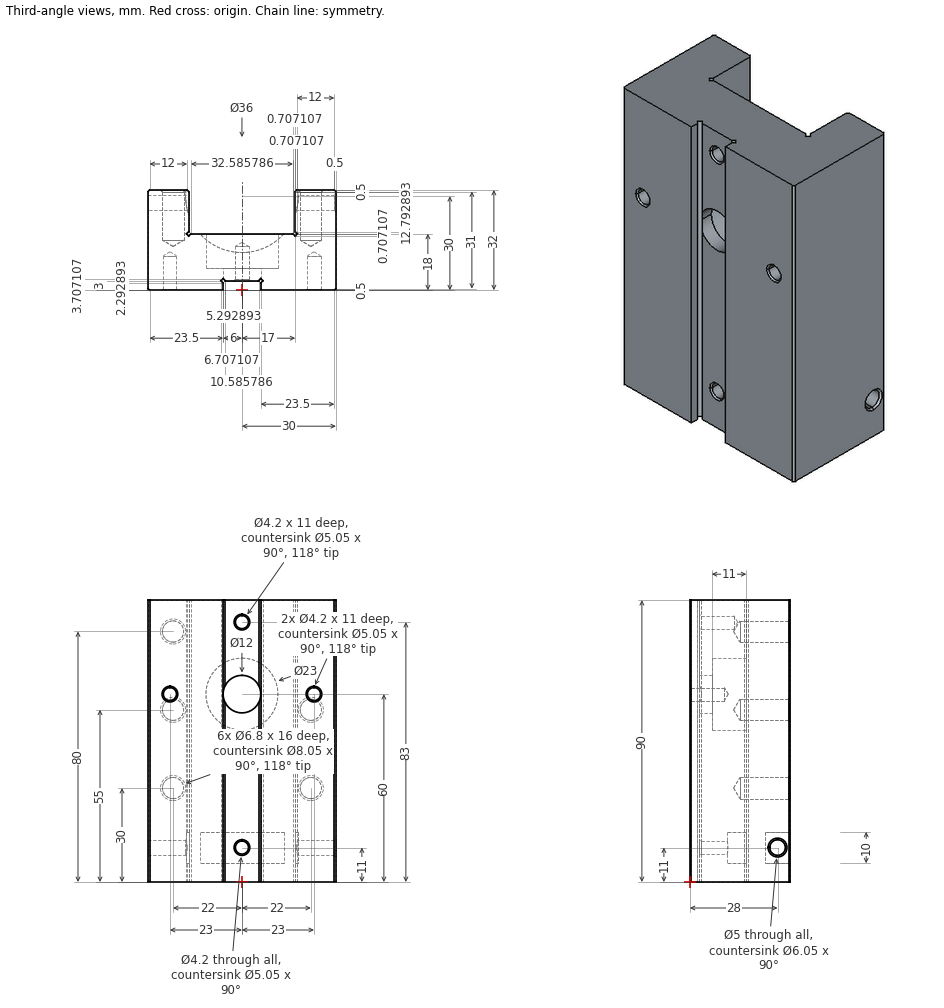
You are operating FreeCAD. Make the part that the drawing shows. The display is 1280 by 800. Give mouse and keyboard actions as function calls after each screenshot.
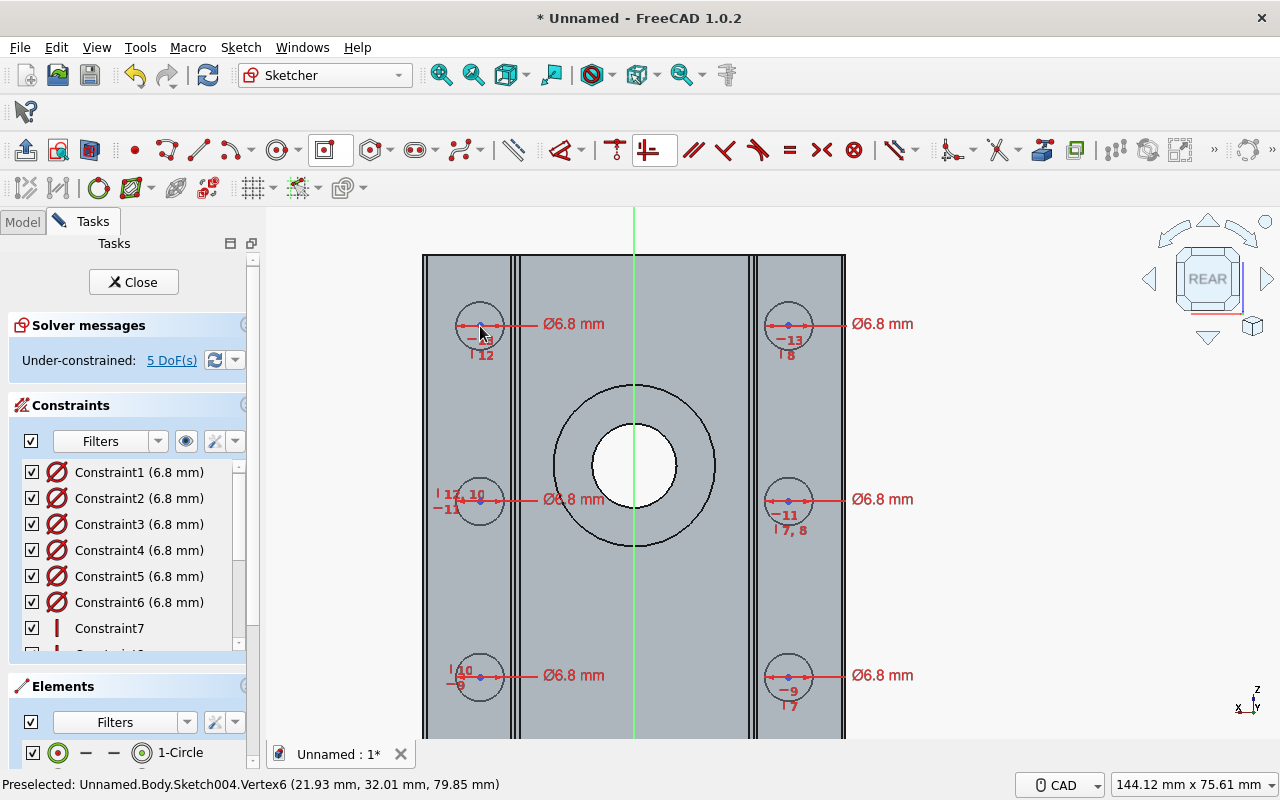
click(560, 150)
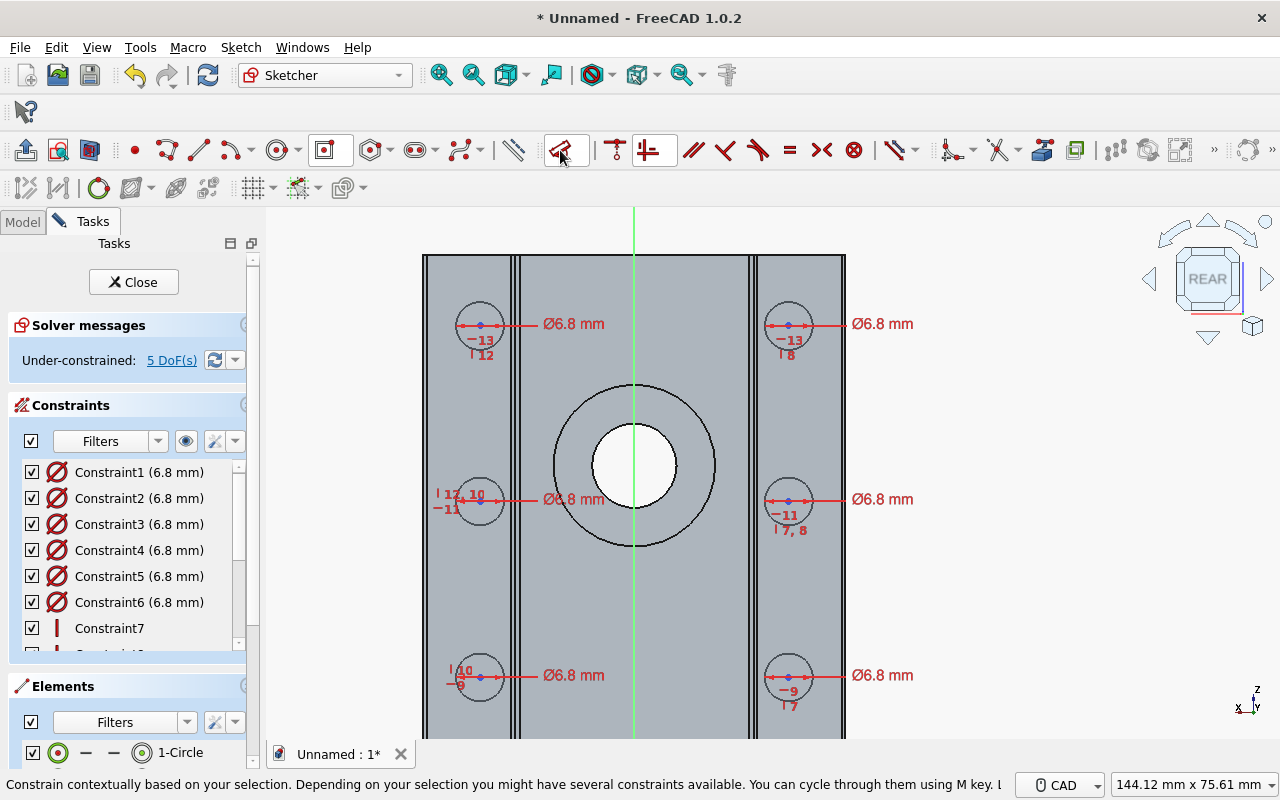
click(789, 677)
click(712, 643)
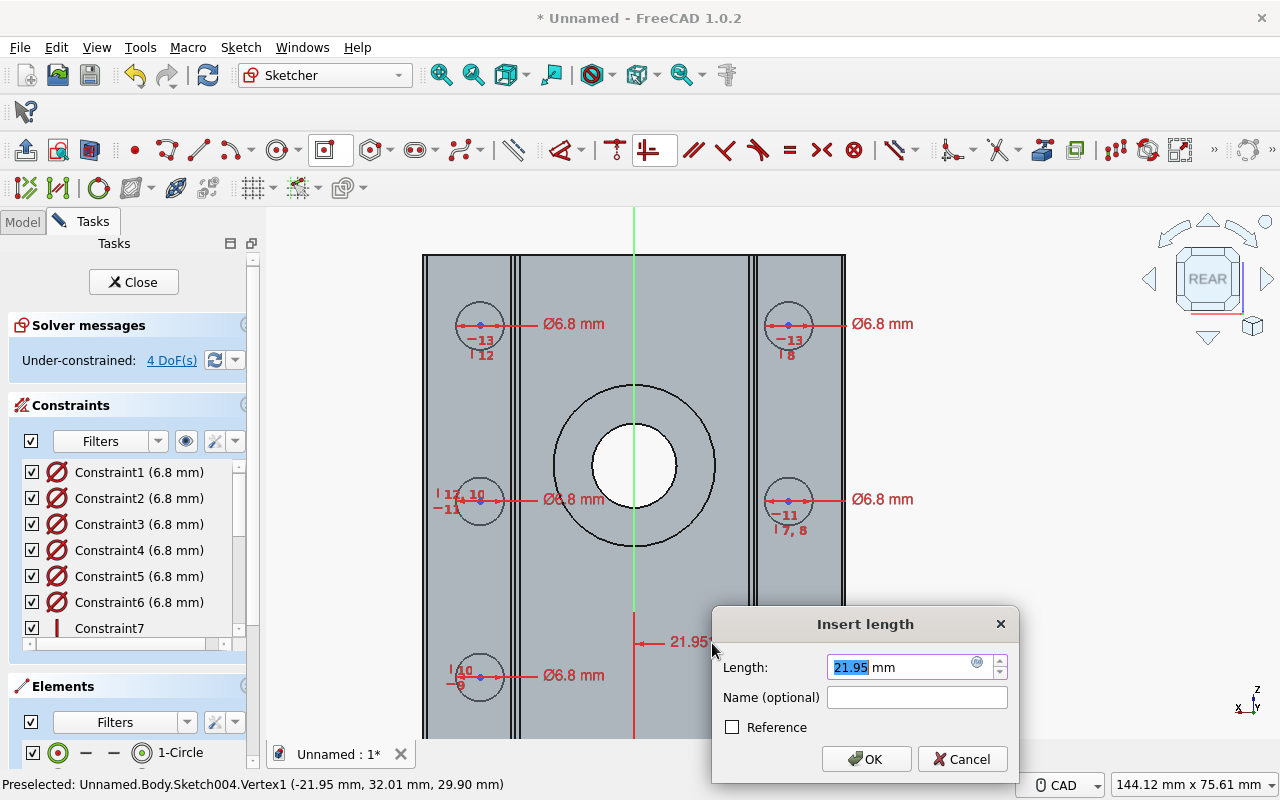
text(22)
key(Return)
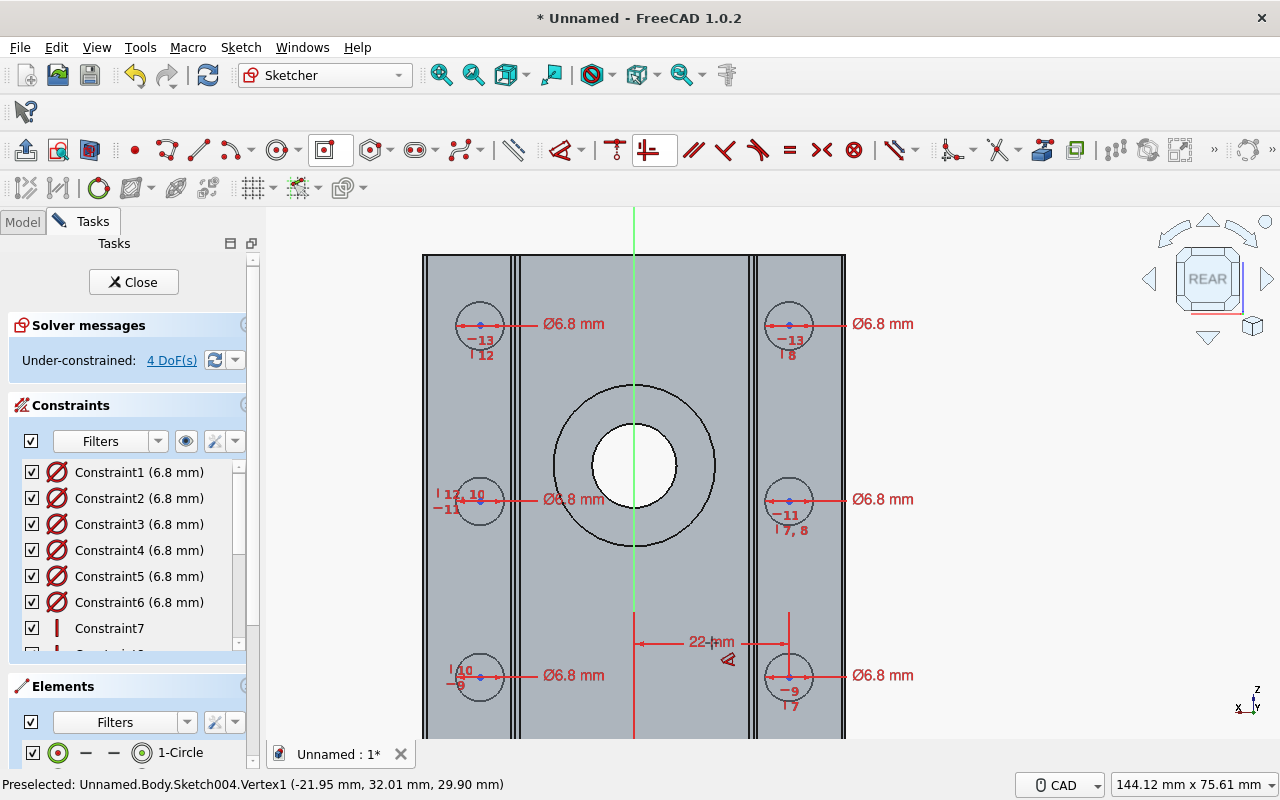
click(789, 677)
click(823, 694)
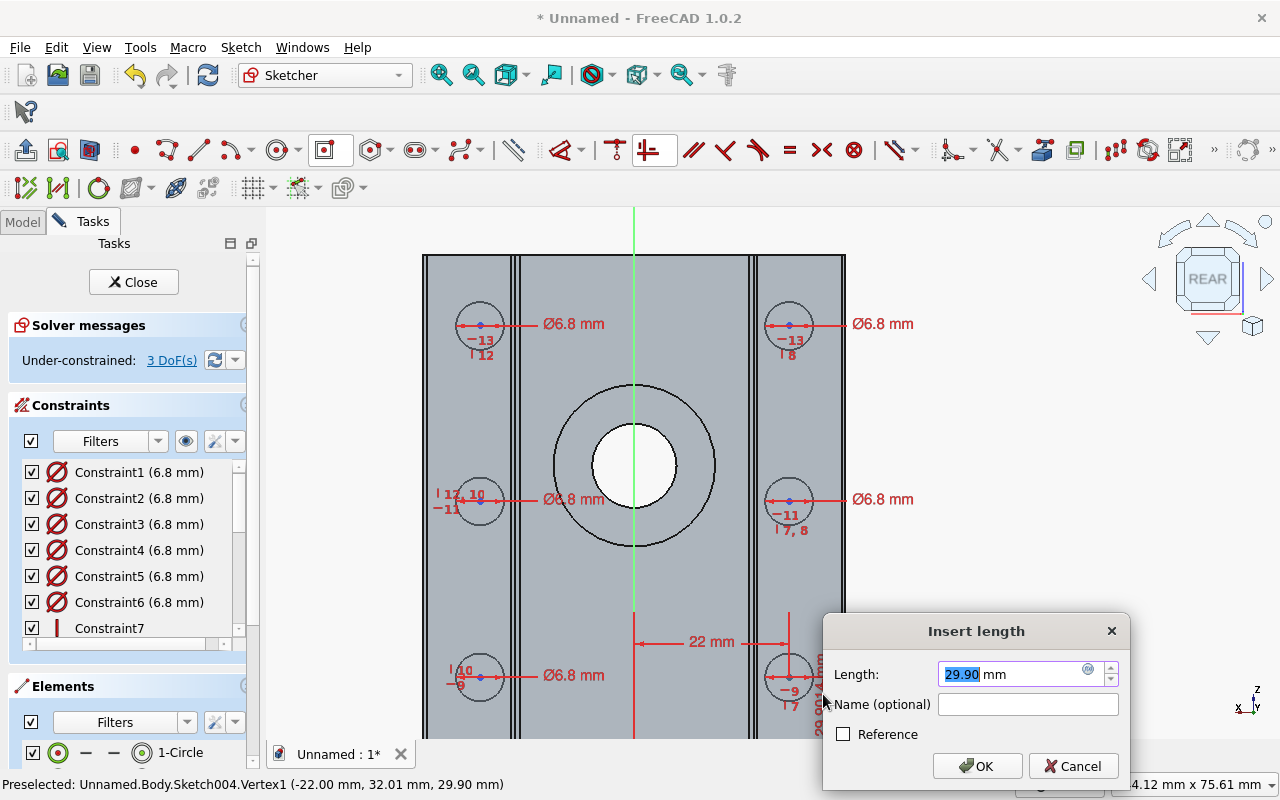
text(30)
key(Return)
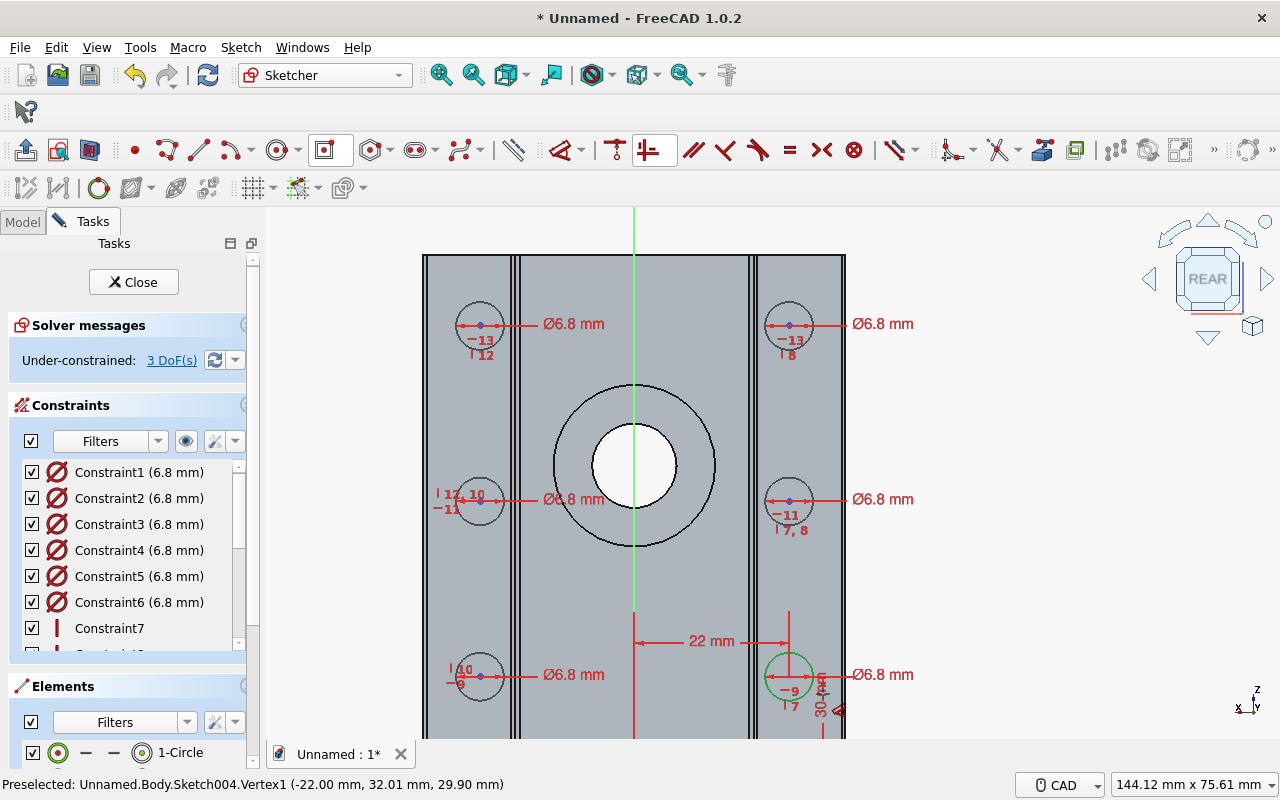
click(789, 501)
click(823, 606)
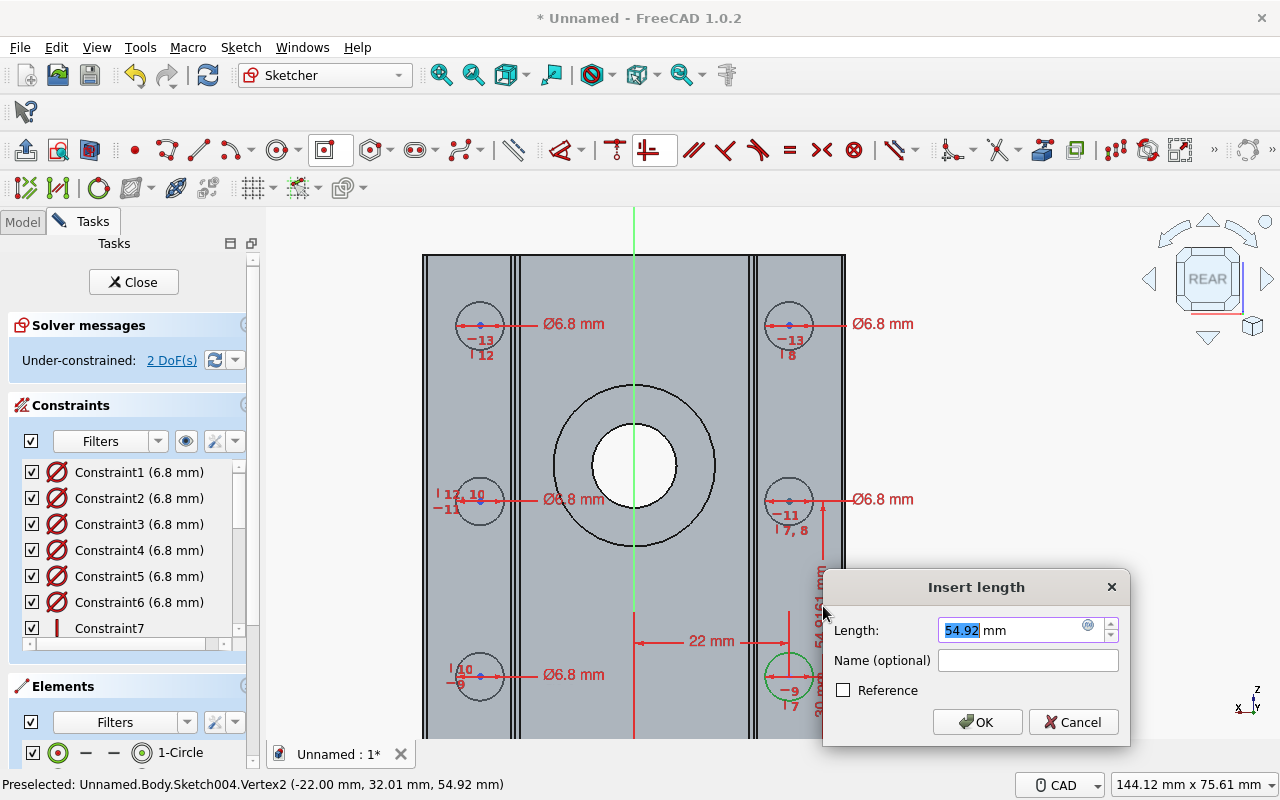
text(55)
key(Return)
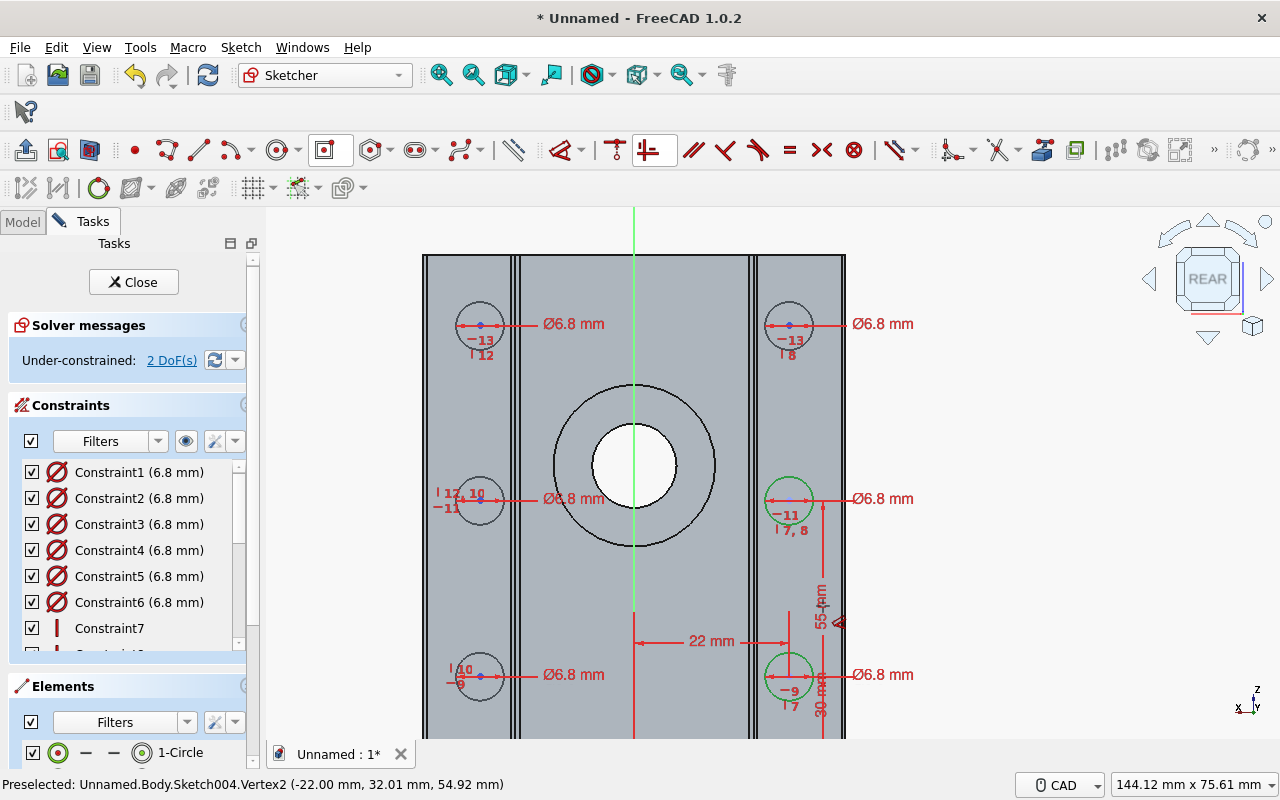
click(789, 326)
click(823, 519)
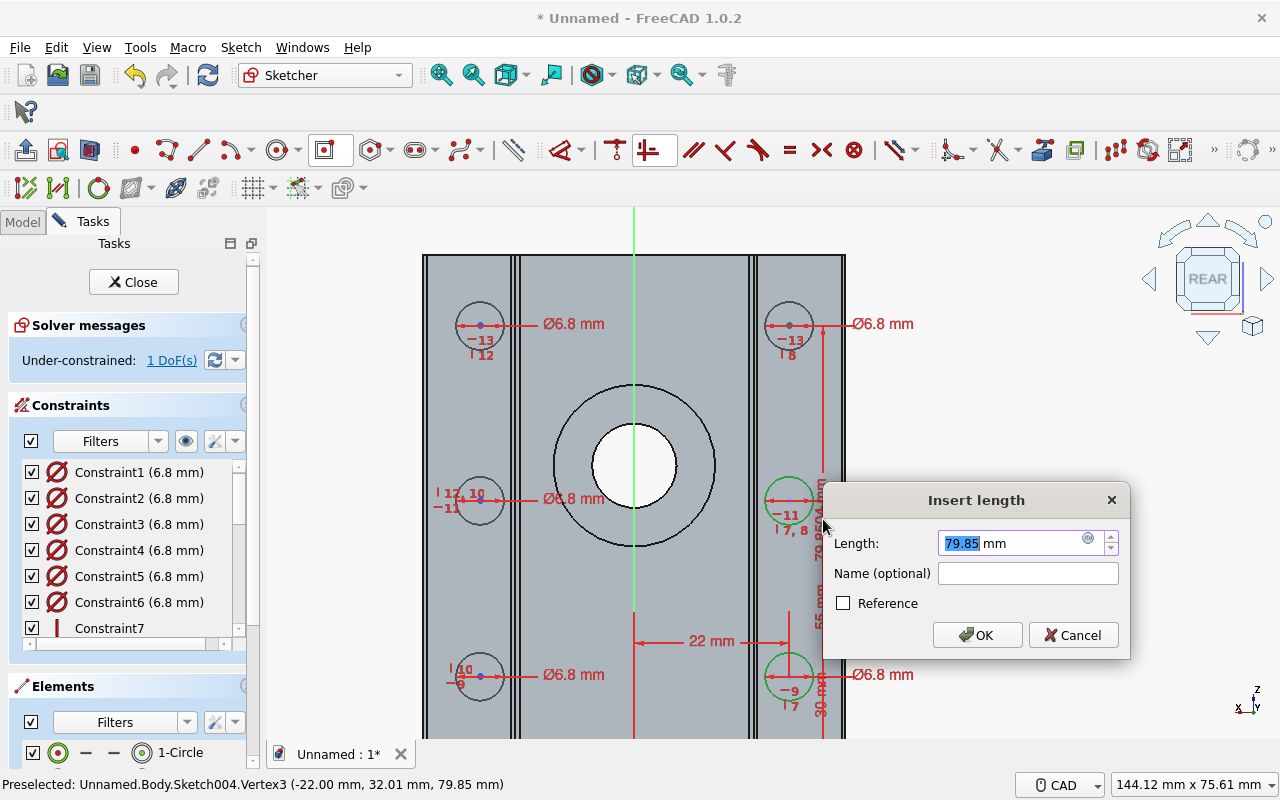
text(80)
key(Return)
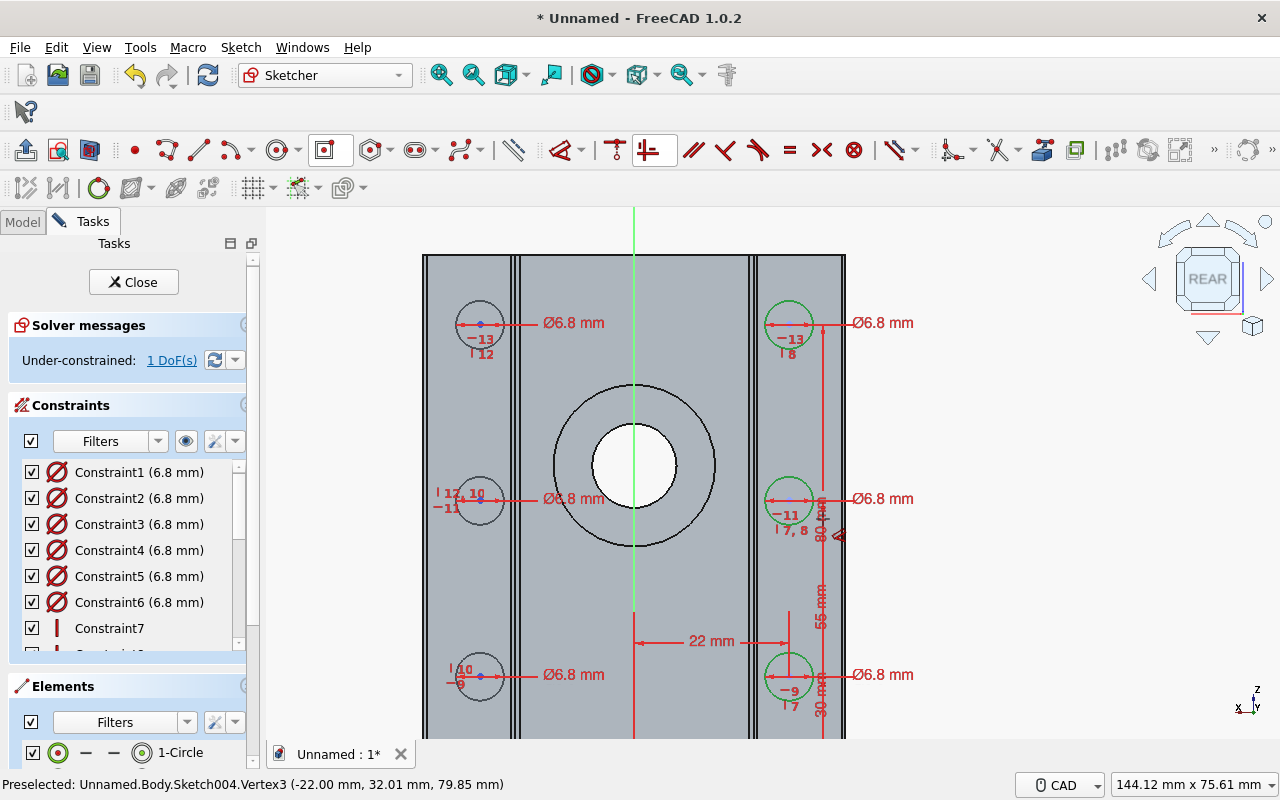
click(480, 677)
click(557, 643)